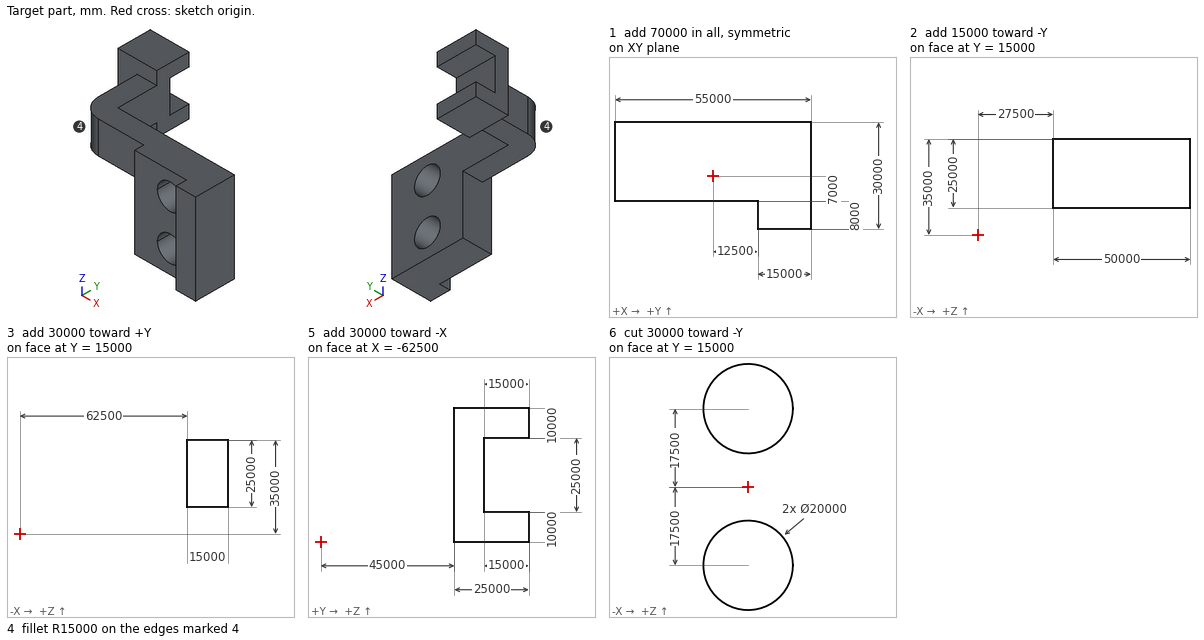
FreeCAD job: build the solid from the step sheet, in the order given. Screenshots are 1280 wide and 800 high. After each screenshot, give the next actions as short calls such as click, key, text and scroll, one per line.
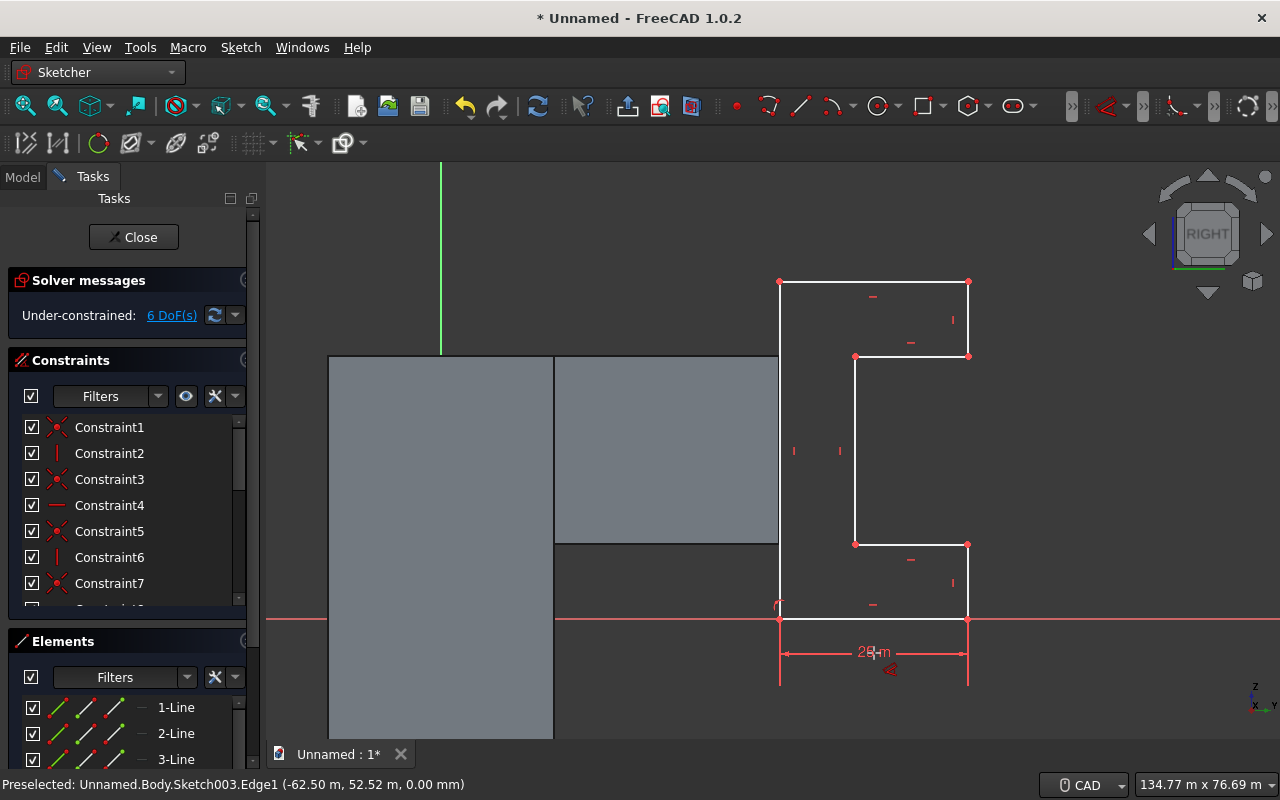
click(968, 597)
click(1002, 582)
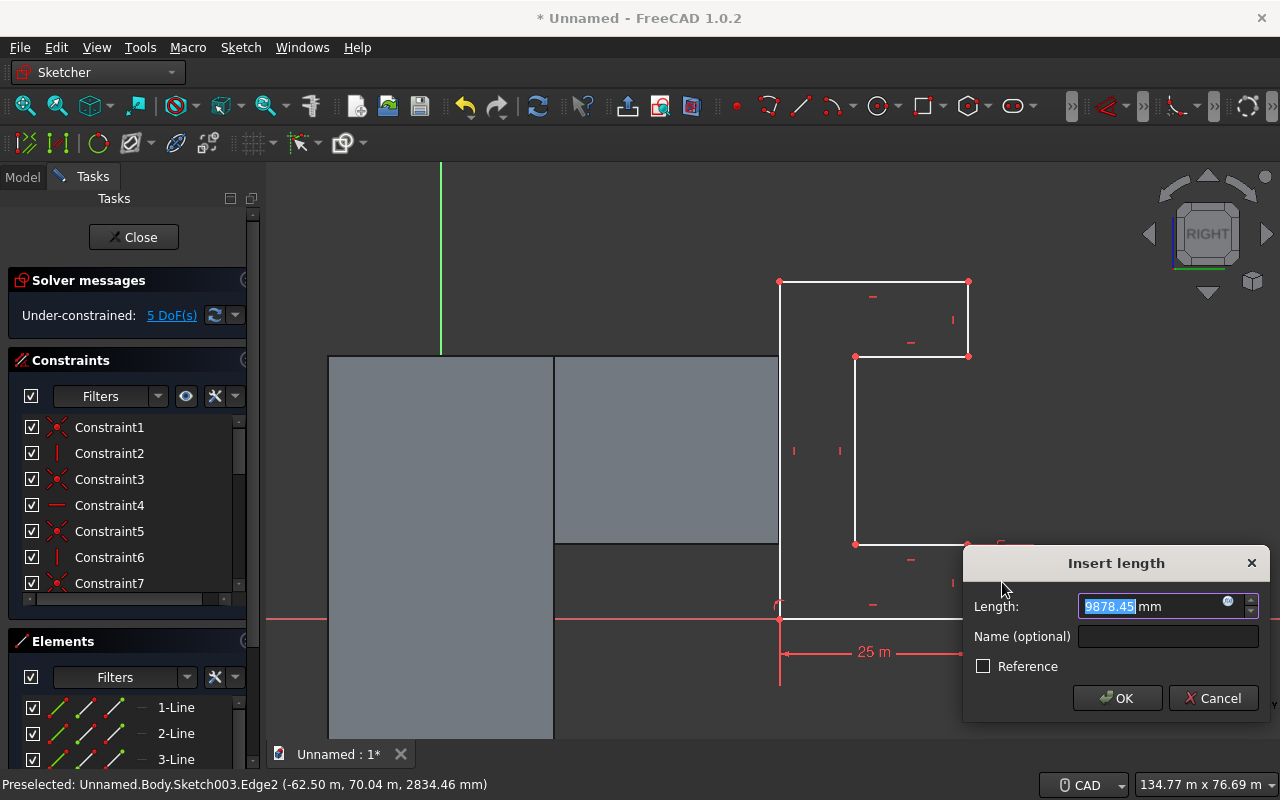
text(10000)
key(Return)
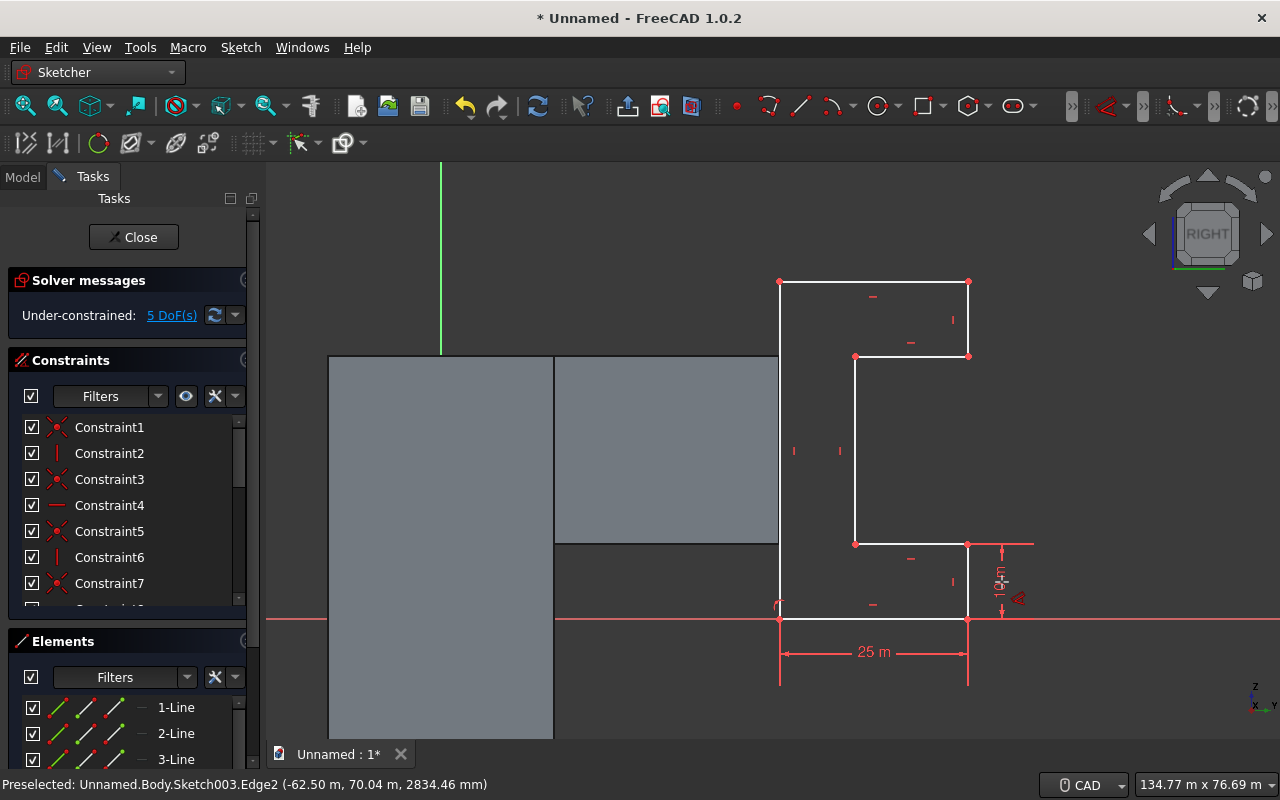
click(934, 544)
click(911, 578)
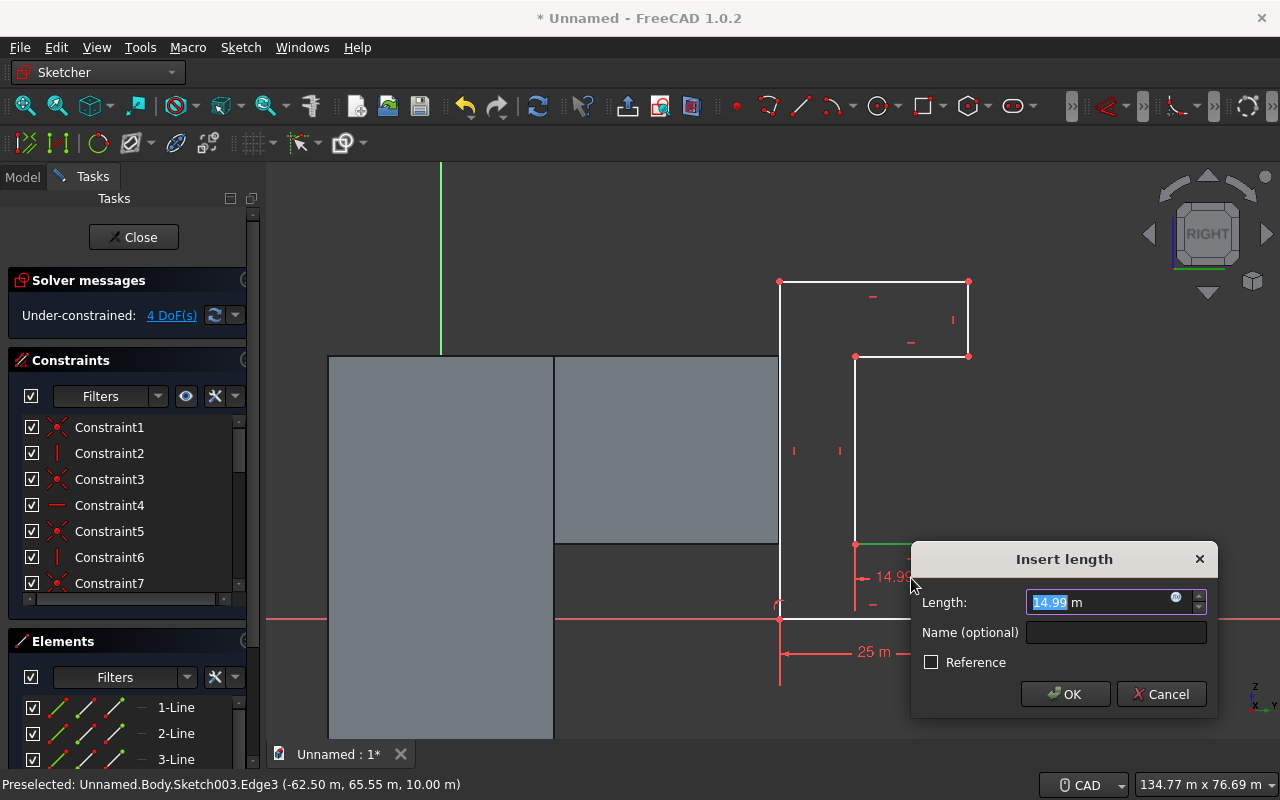
key(ctrl+a)
text(15000 mm)
key(Return)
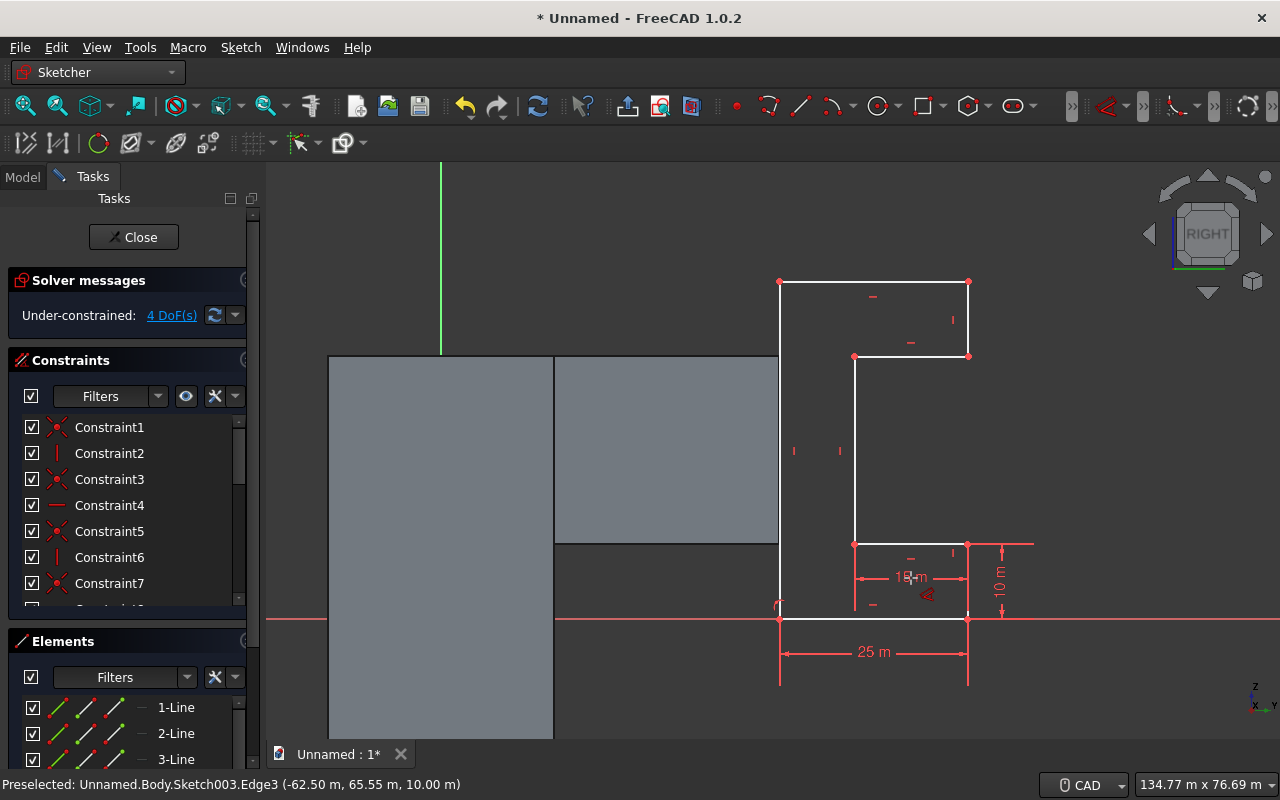
click(855, 488)
click(889, 451)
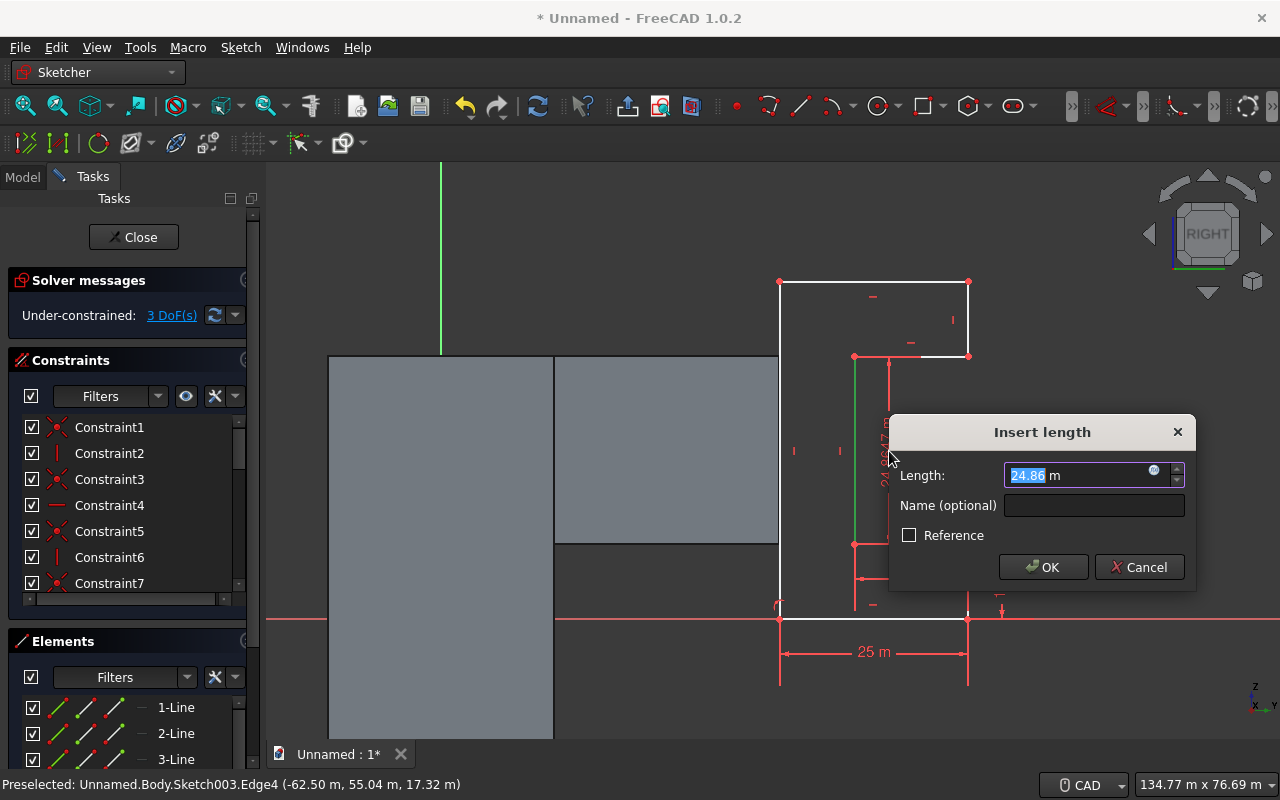
key(ctrl+a)
text(25000 mm)
key(Return)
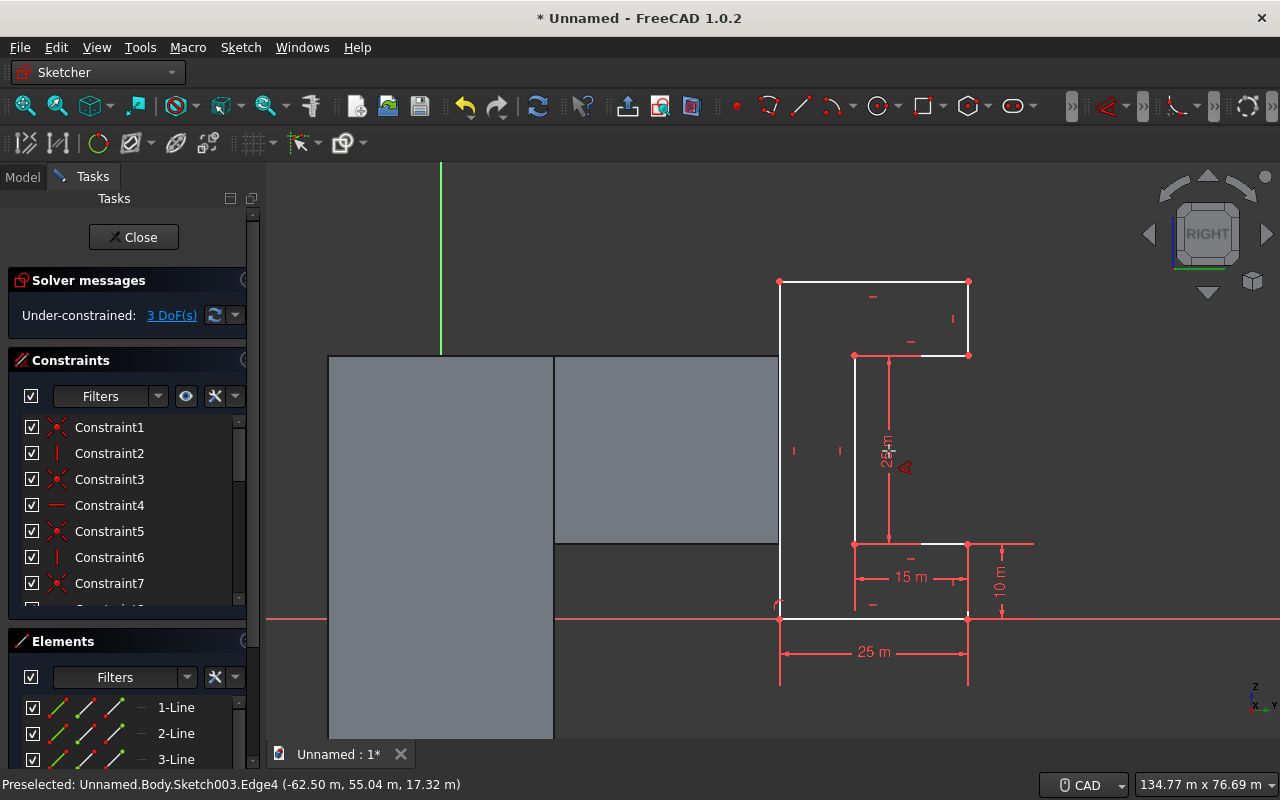
click(889, 356)
click(911, 322)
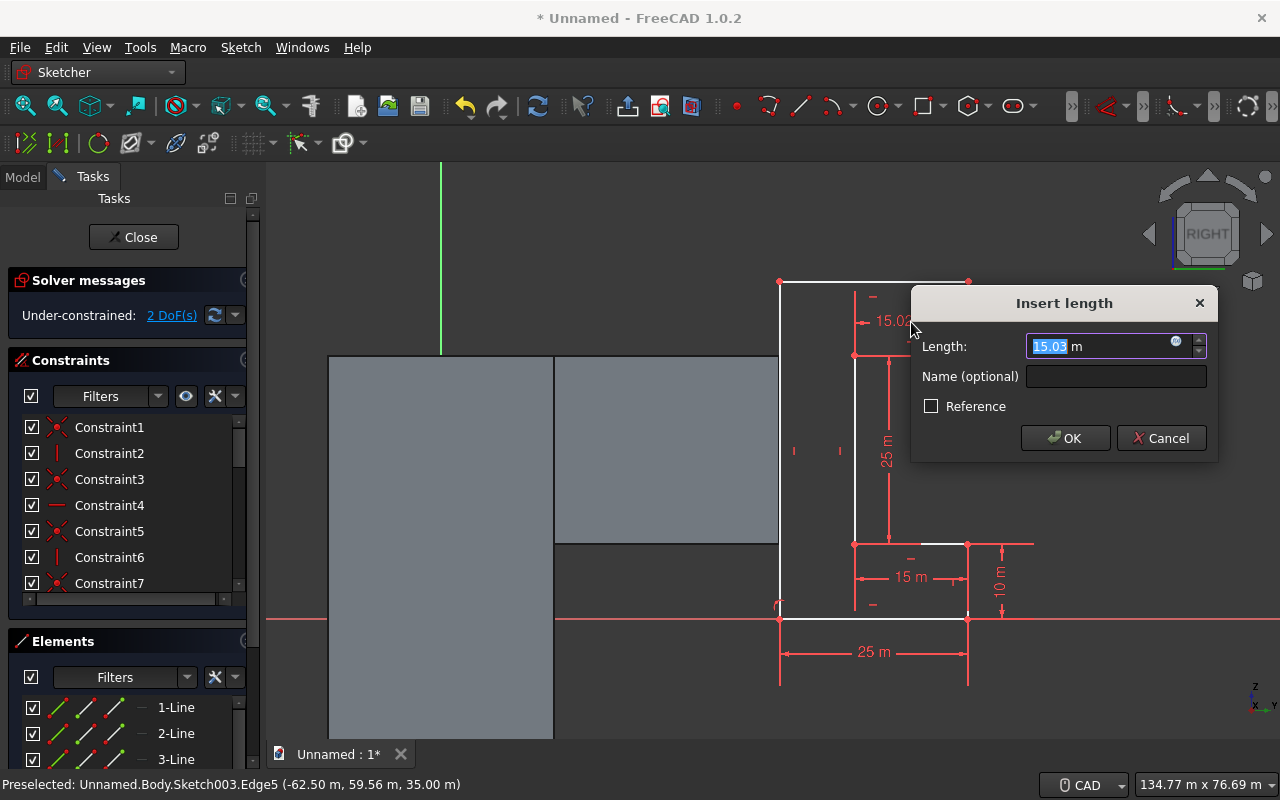
key(ctrl+a)
text(15000 mm)
key(Return)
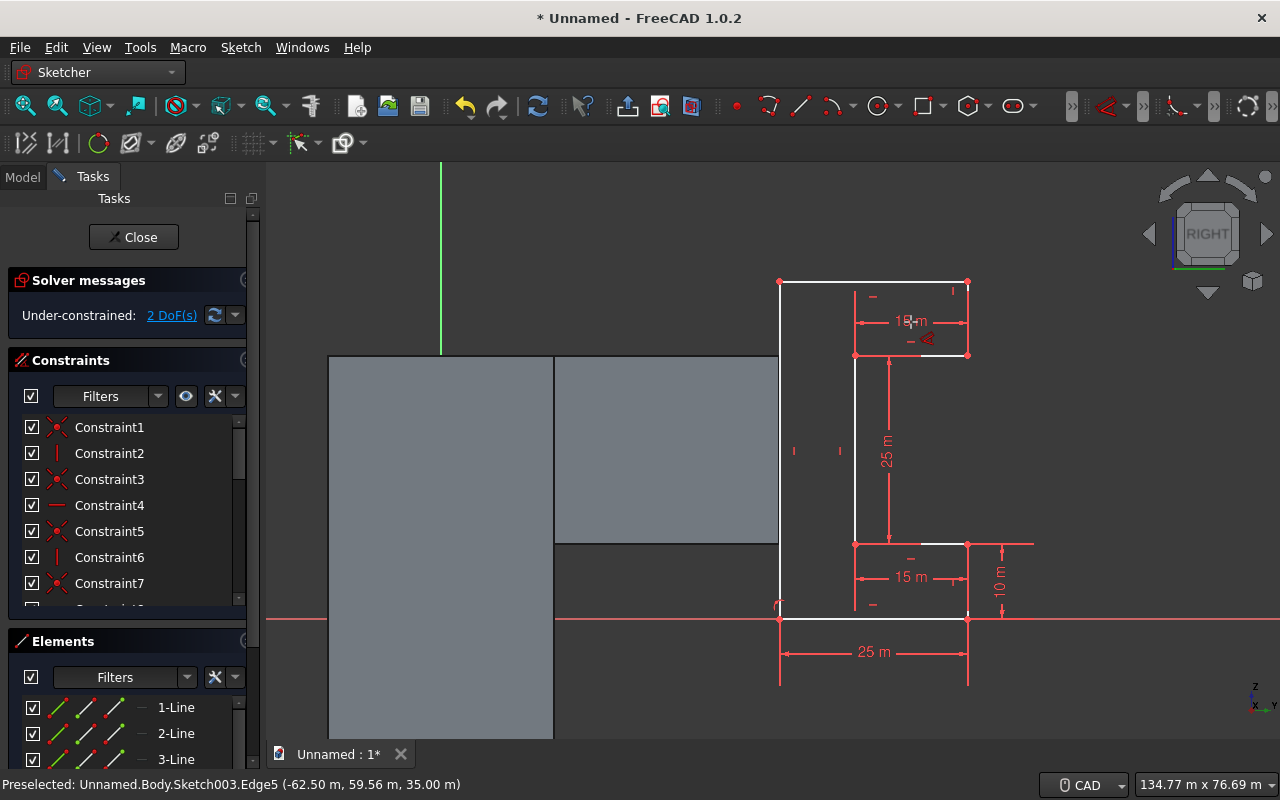
click(968, 334)
click(1002, 319)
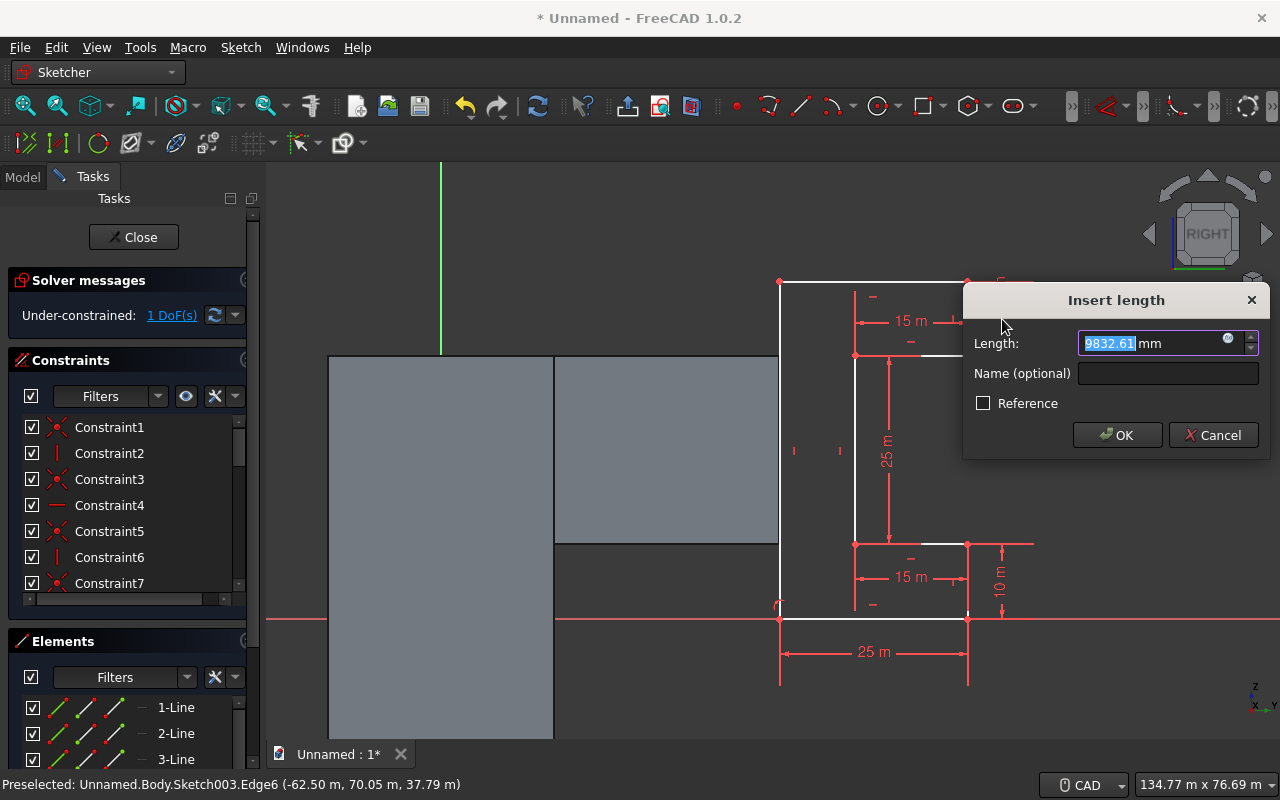
text(10000)
key(Return)